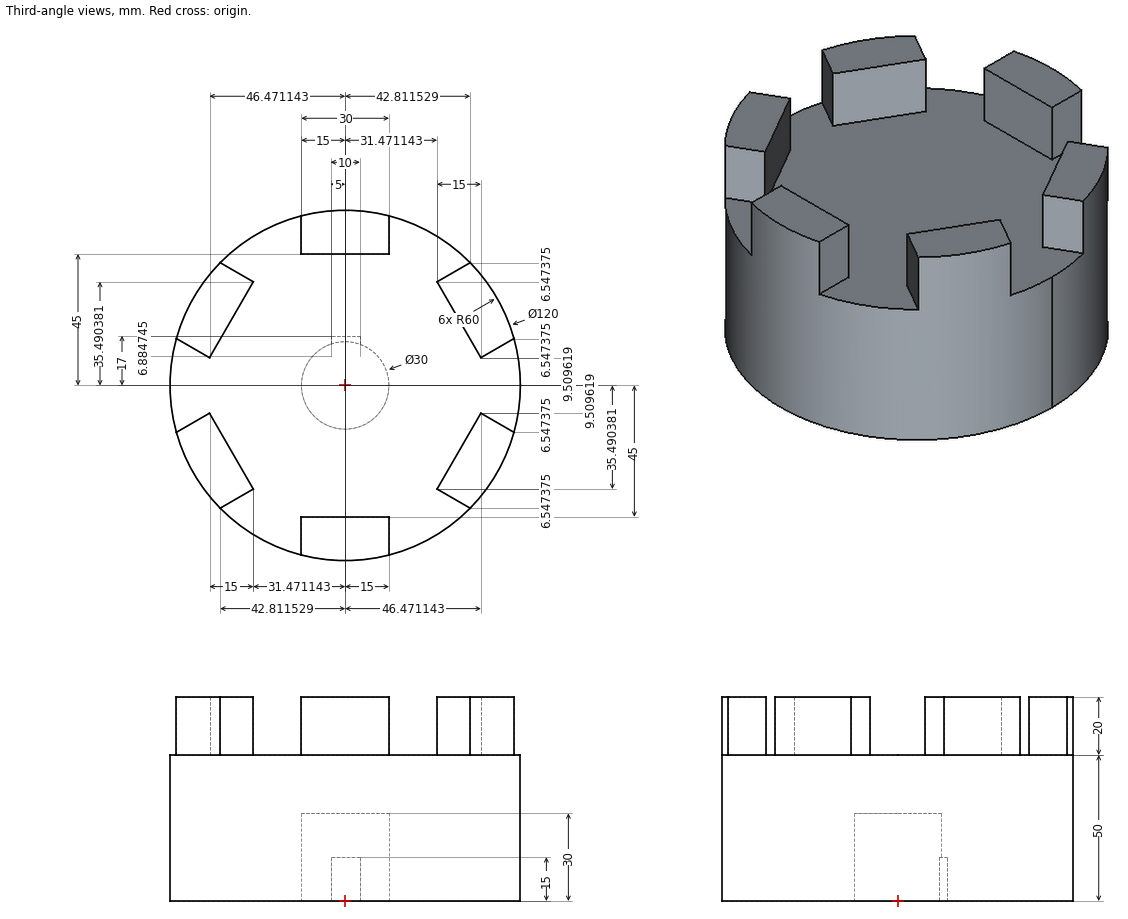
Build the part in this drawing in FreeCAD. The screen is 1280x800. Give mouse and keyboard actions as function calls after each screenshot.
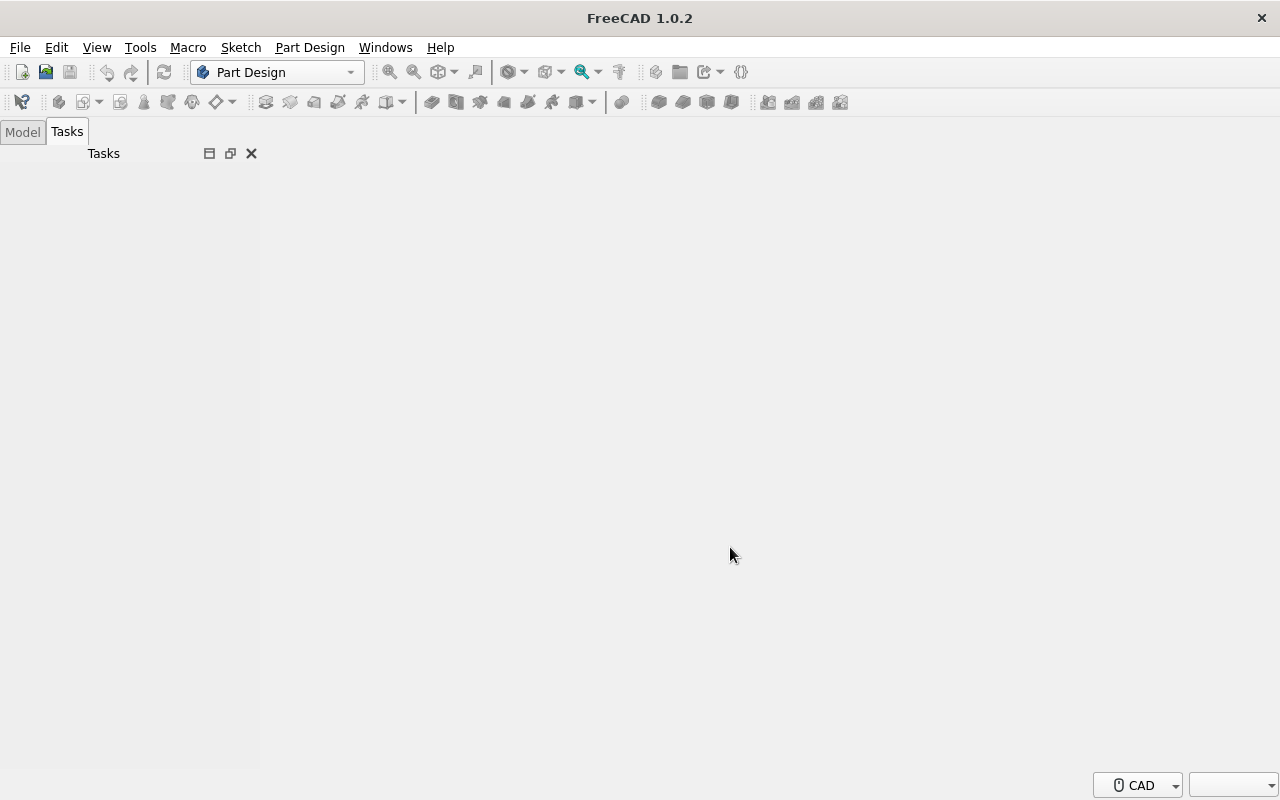
key(ctrl+n)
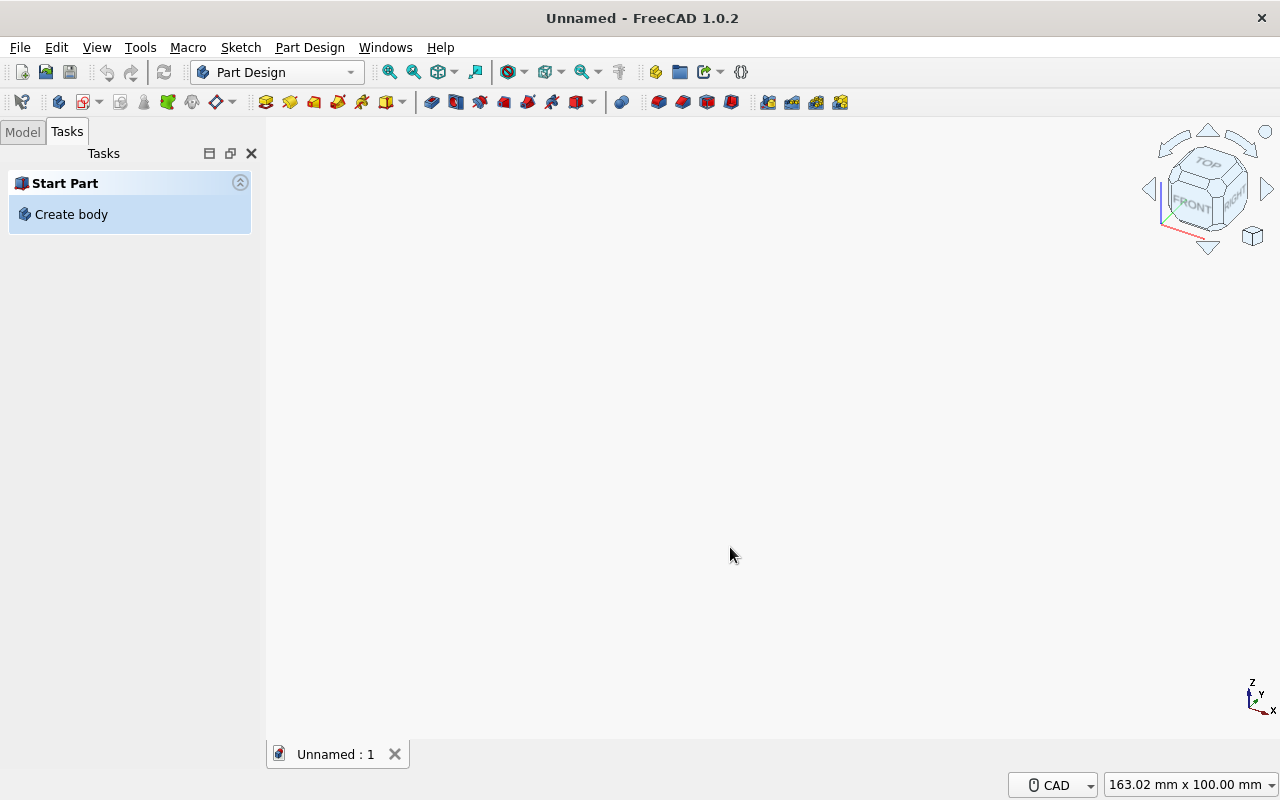
click(84, 102)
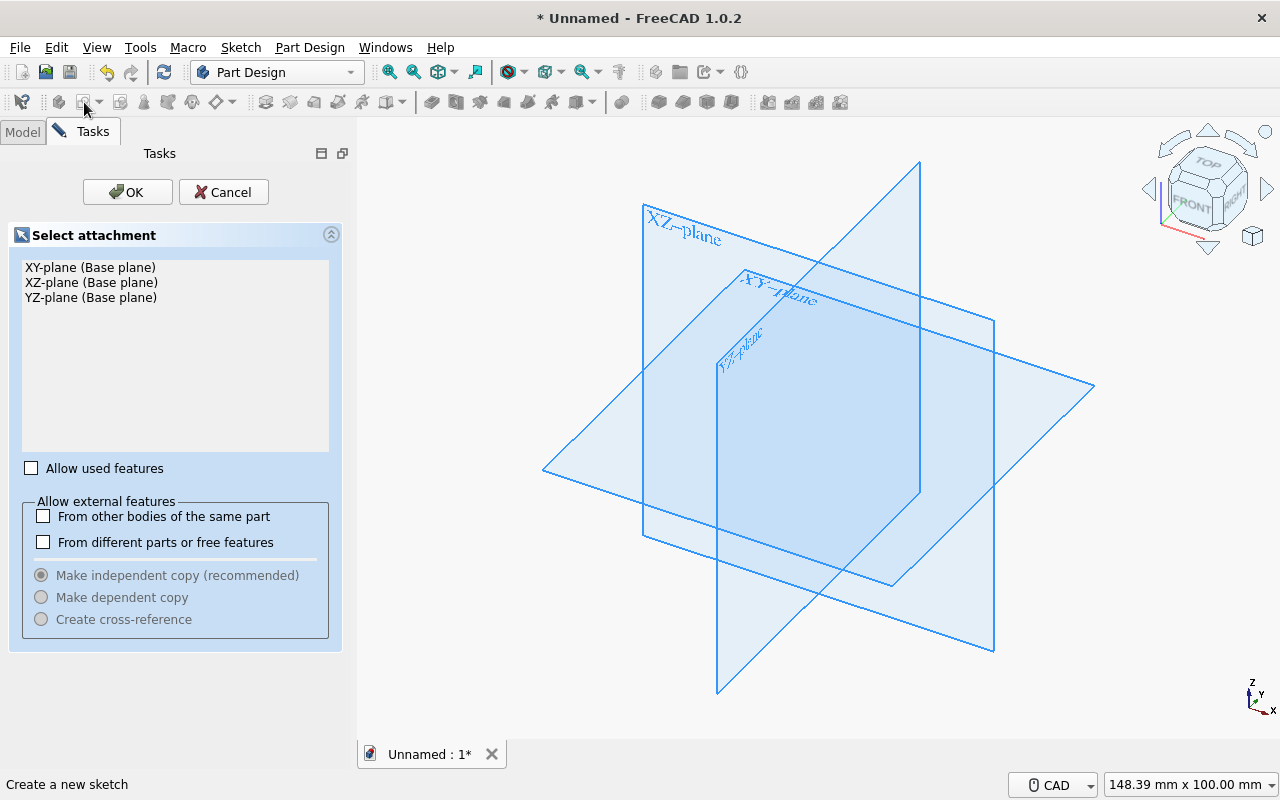
click(82, 268)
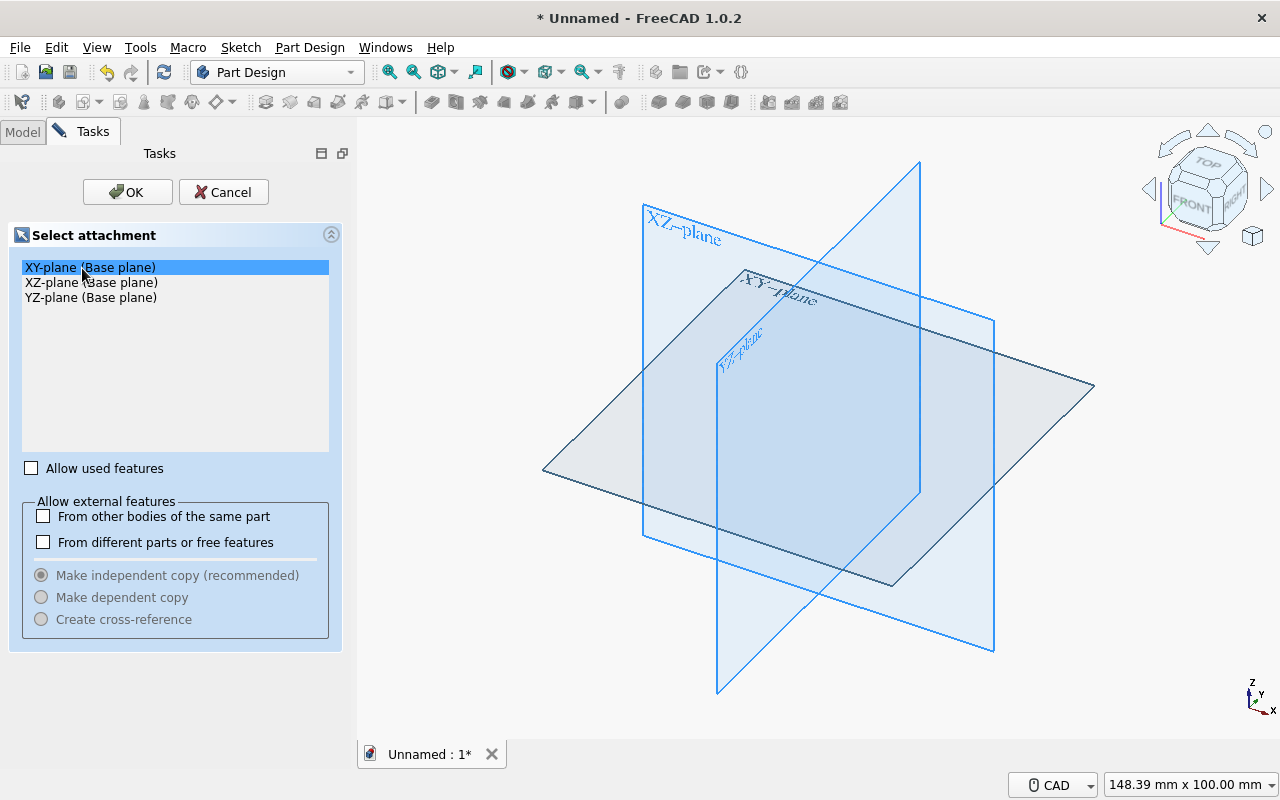
click(128, 192)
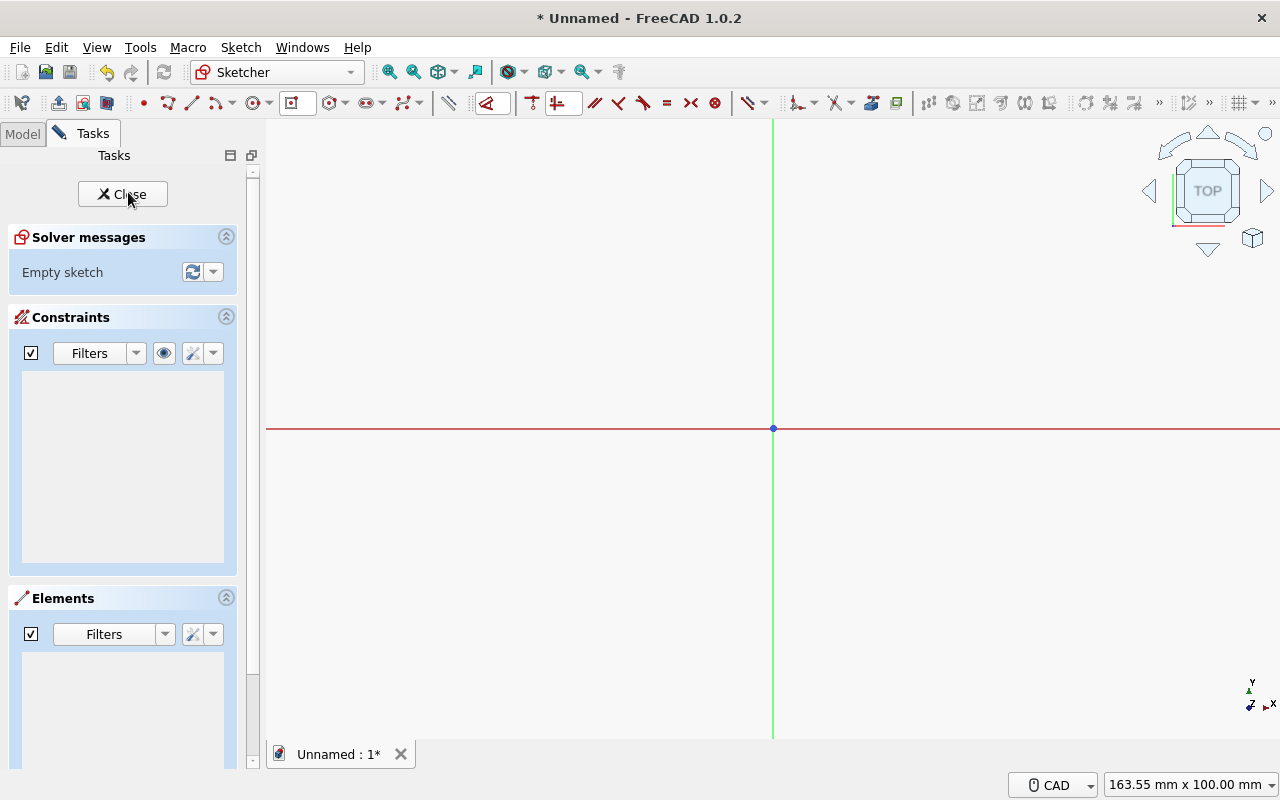
scroll(621, 429, down, 3)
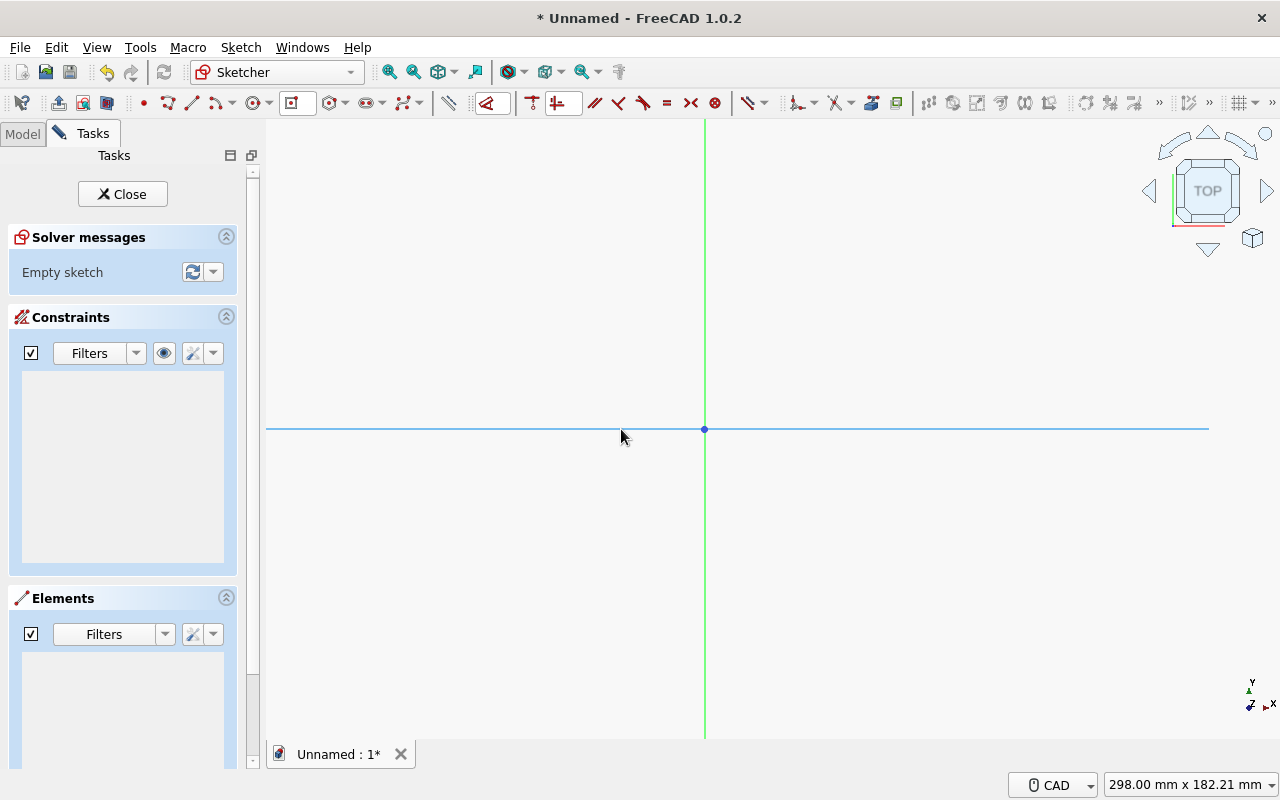
key(g)
key(c)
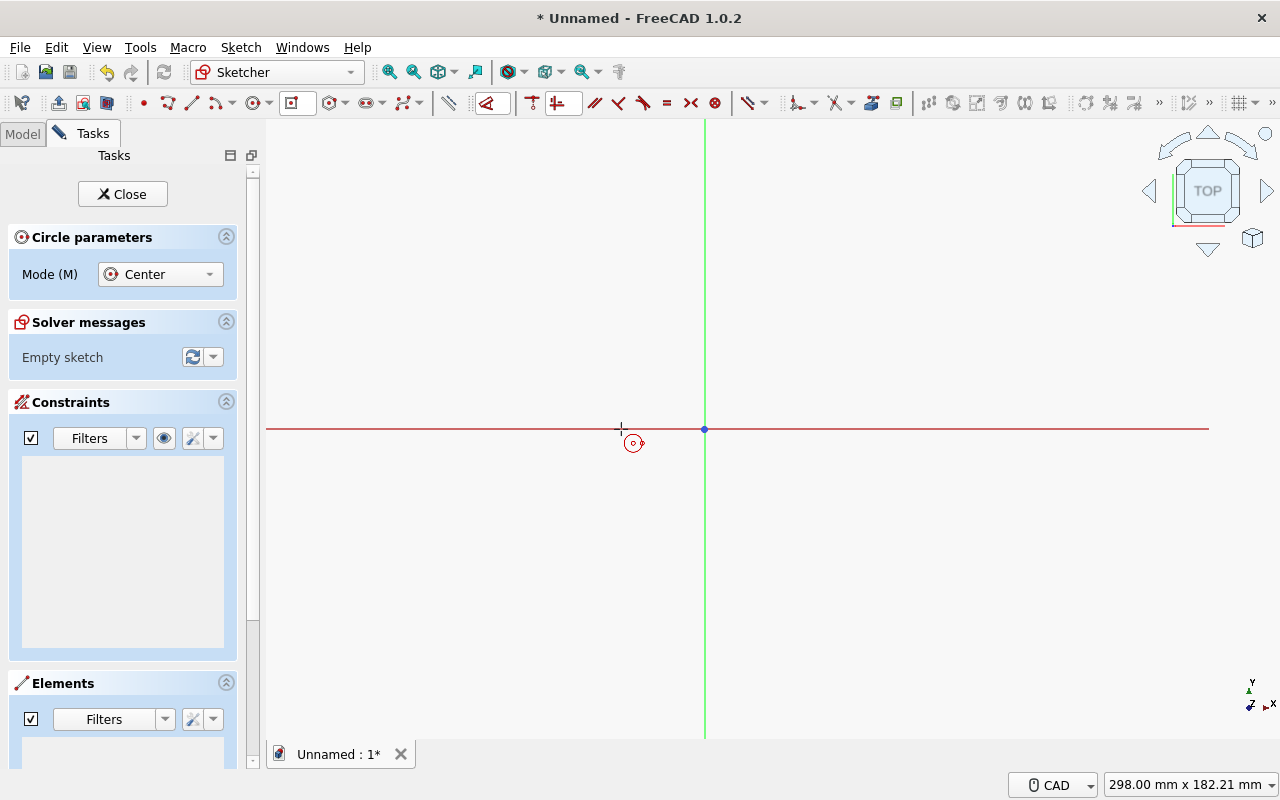
click(705, 429)
click(849, 285)
key(Escape)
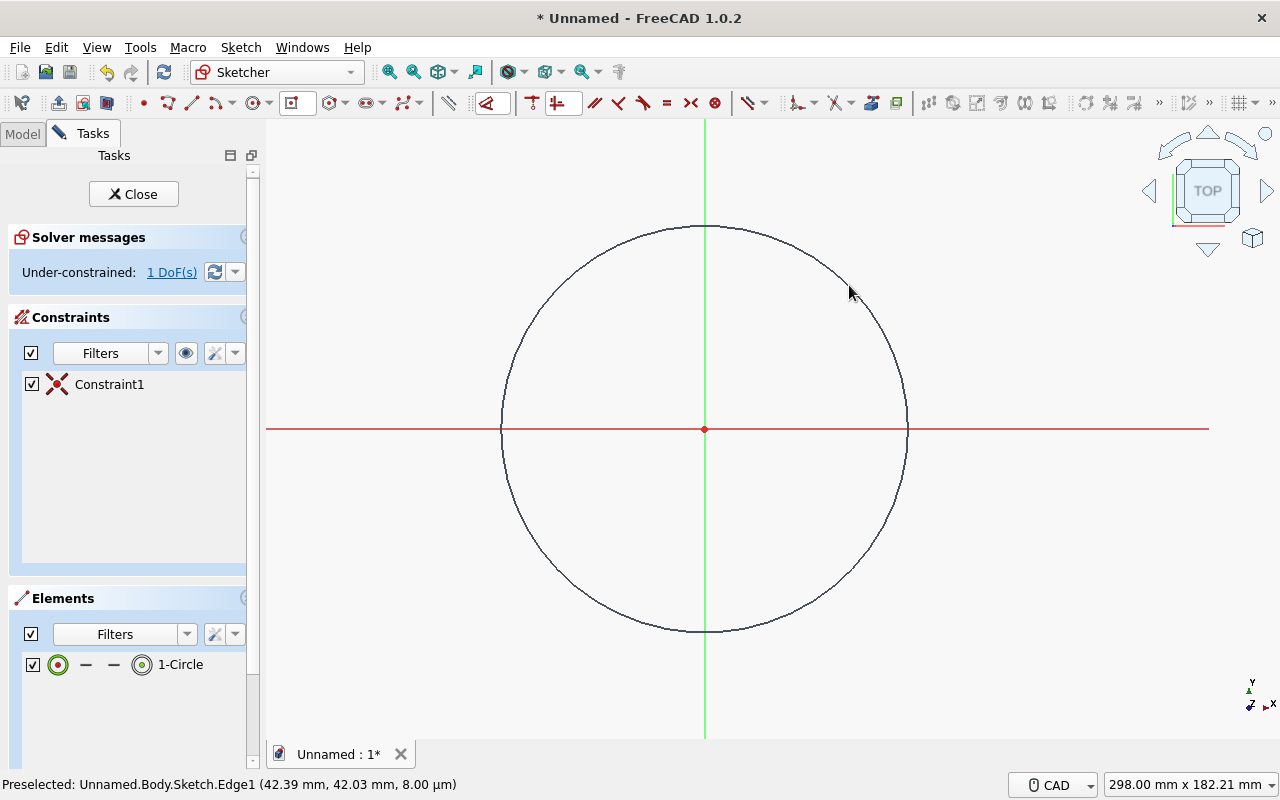
click(848, 285)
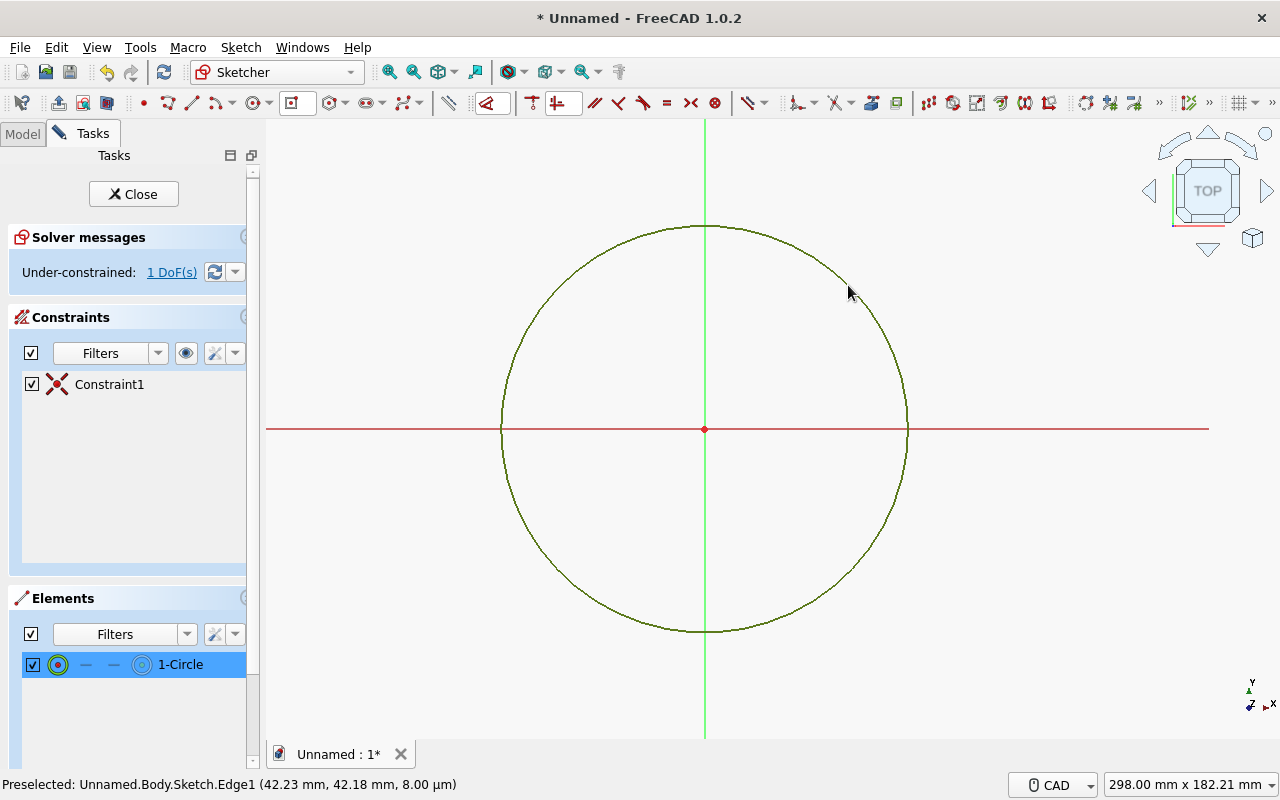
key(k)
key(o)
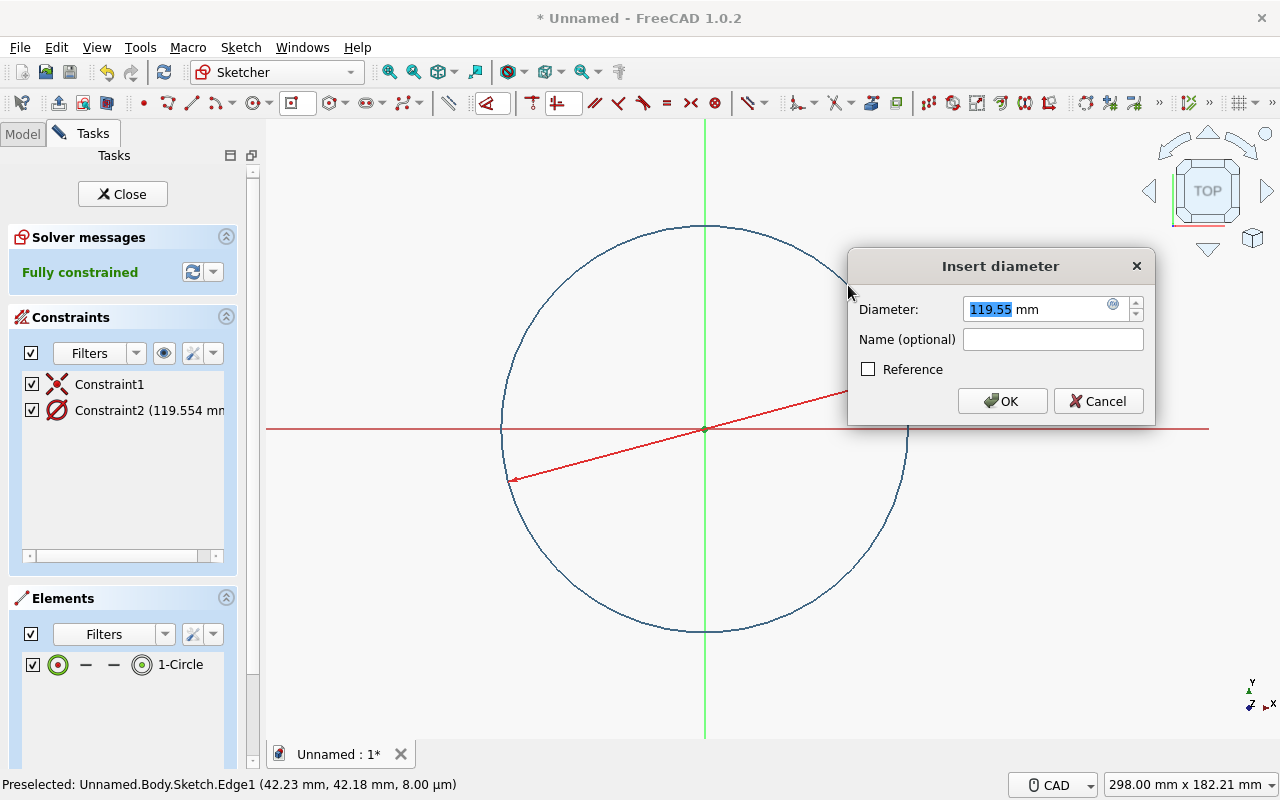
text(120)
key(Return)